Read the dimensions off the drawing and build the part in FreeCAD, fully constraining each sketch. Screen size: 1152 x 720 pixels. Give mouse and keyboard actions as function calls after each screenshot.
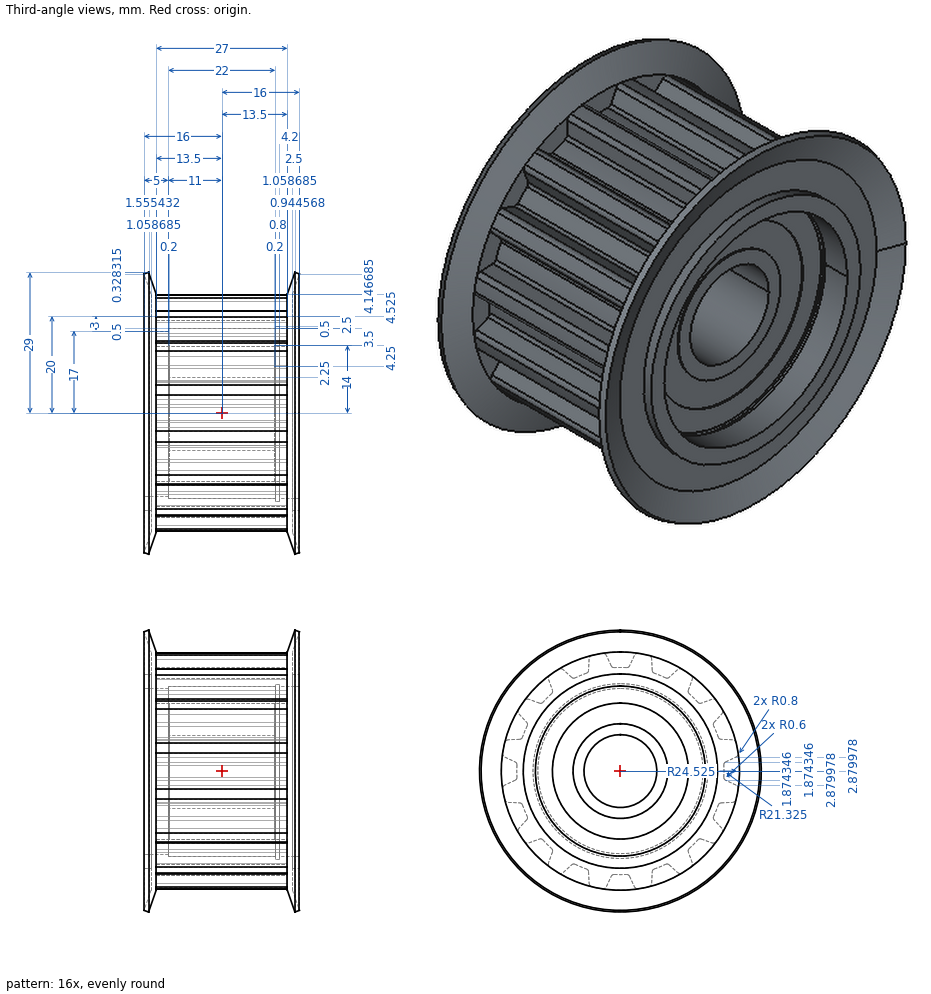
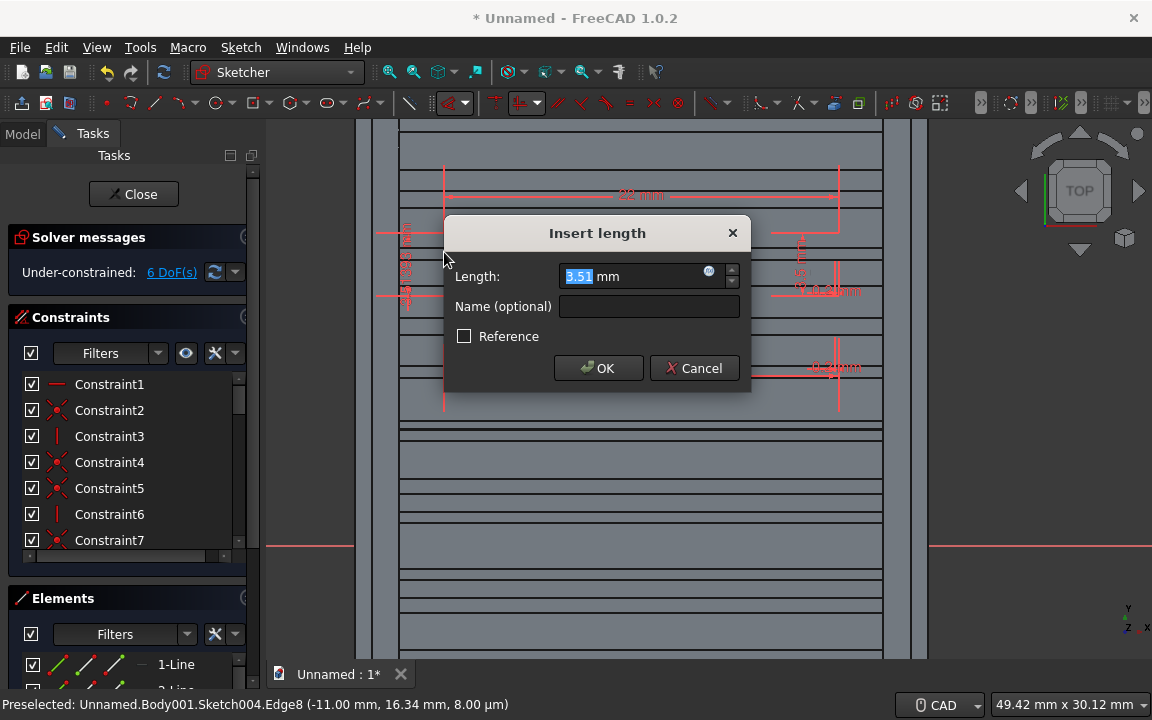
text(3.5)
key(Return)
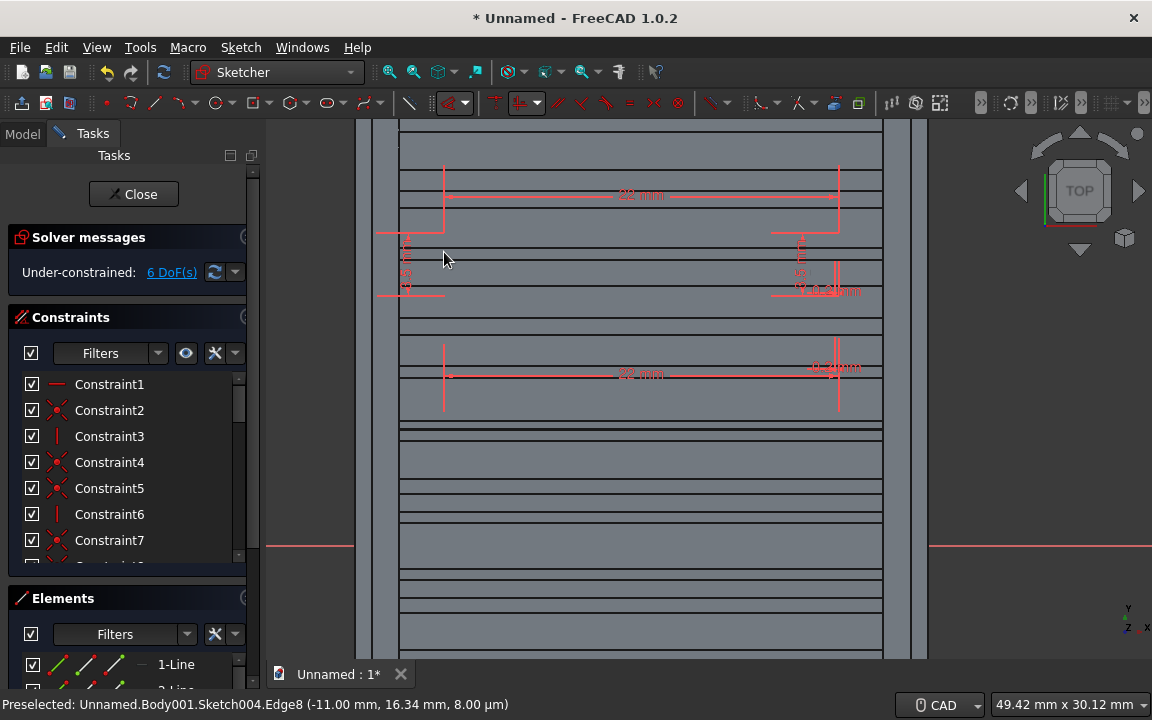
scroll(446, 296, up, 13)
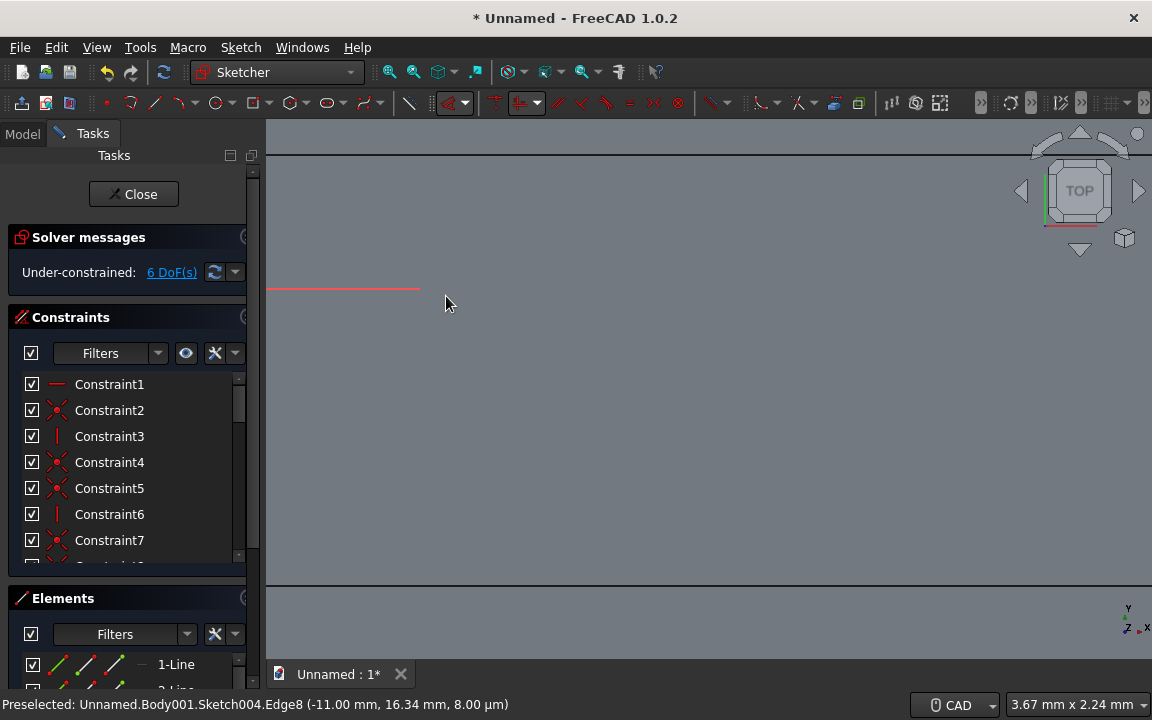
click(444, 289)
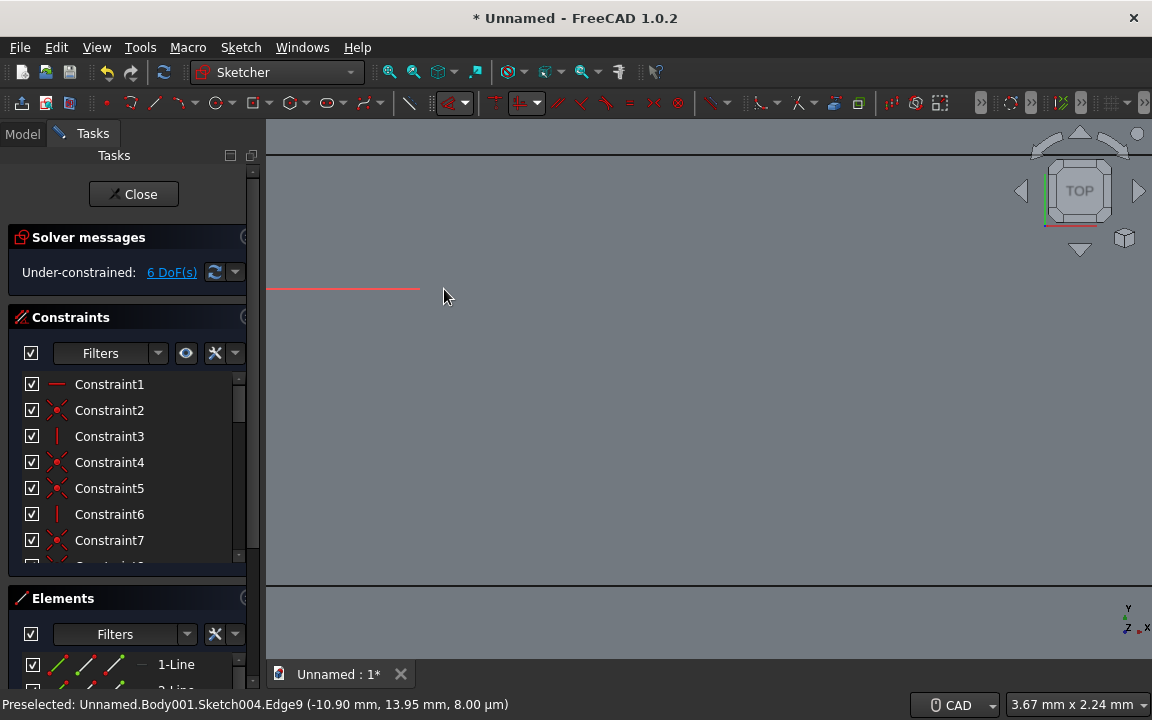
click(468, 104)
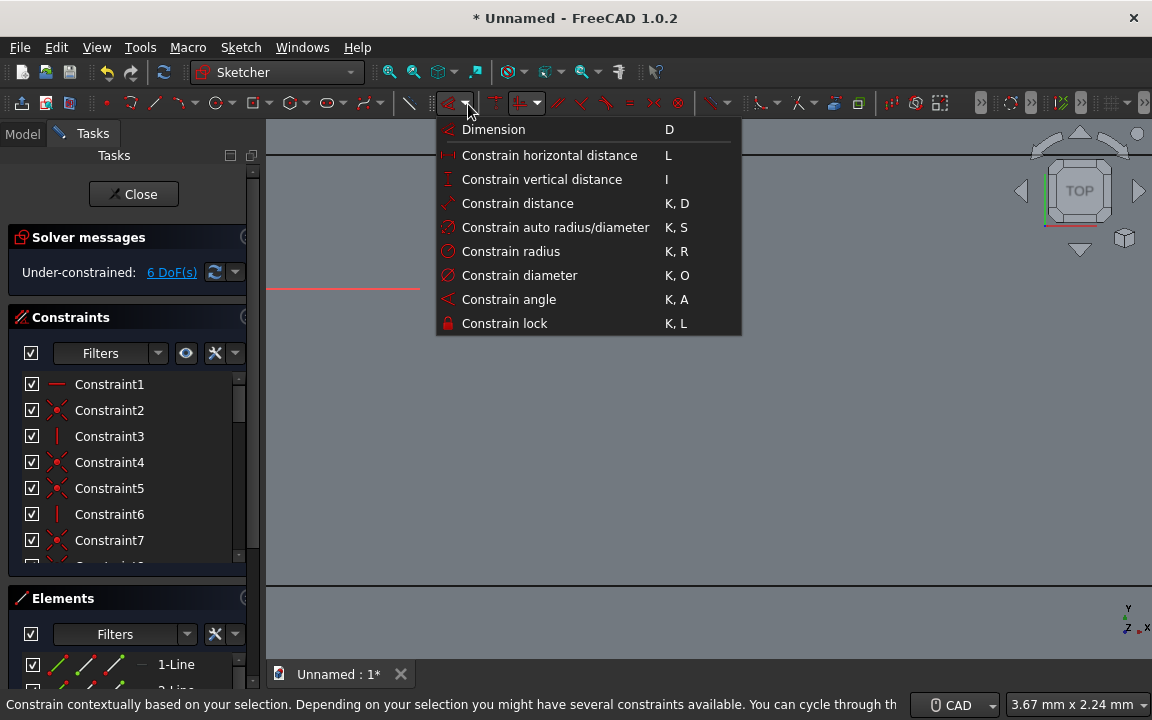
click(589, 155)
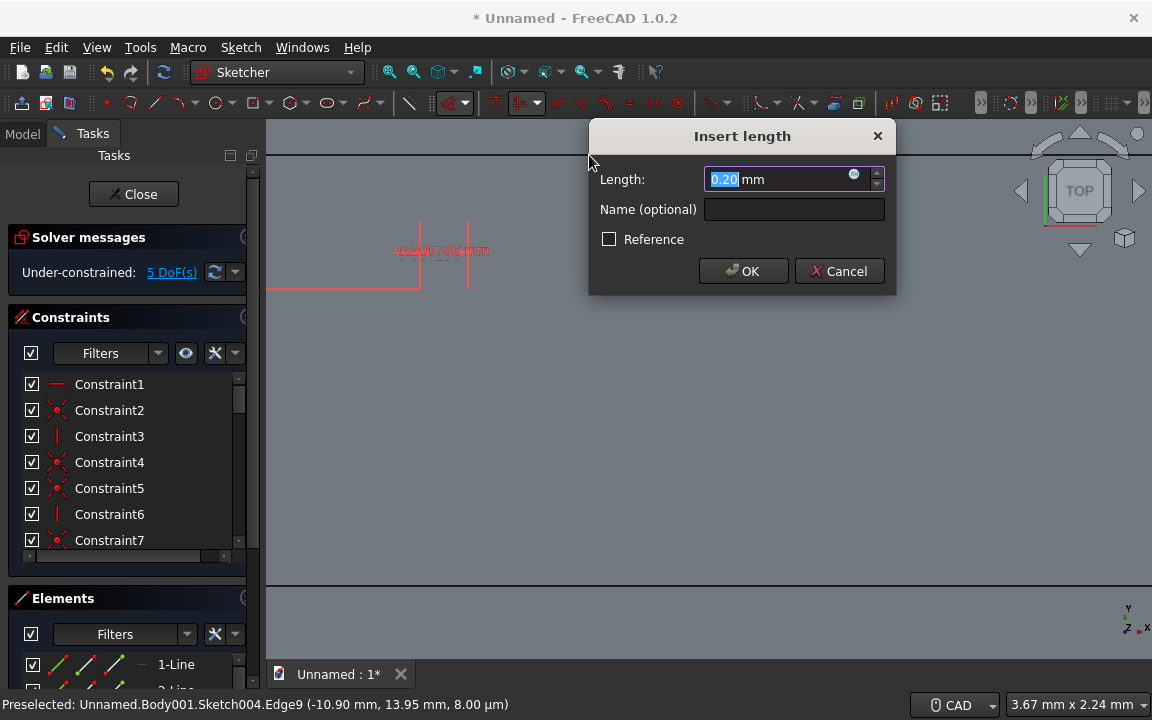
text(0.2)
key(Return)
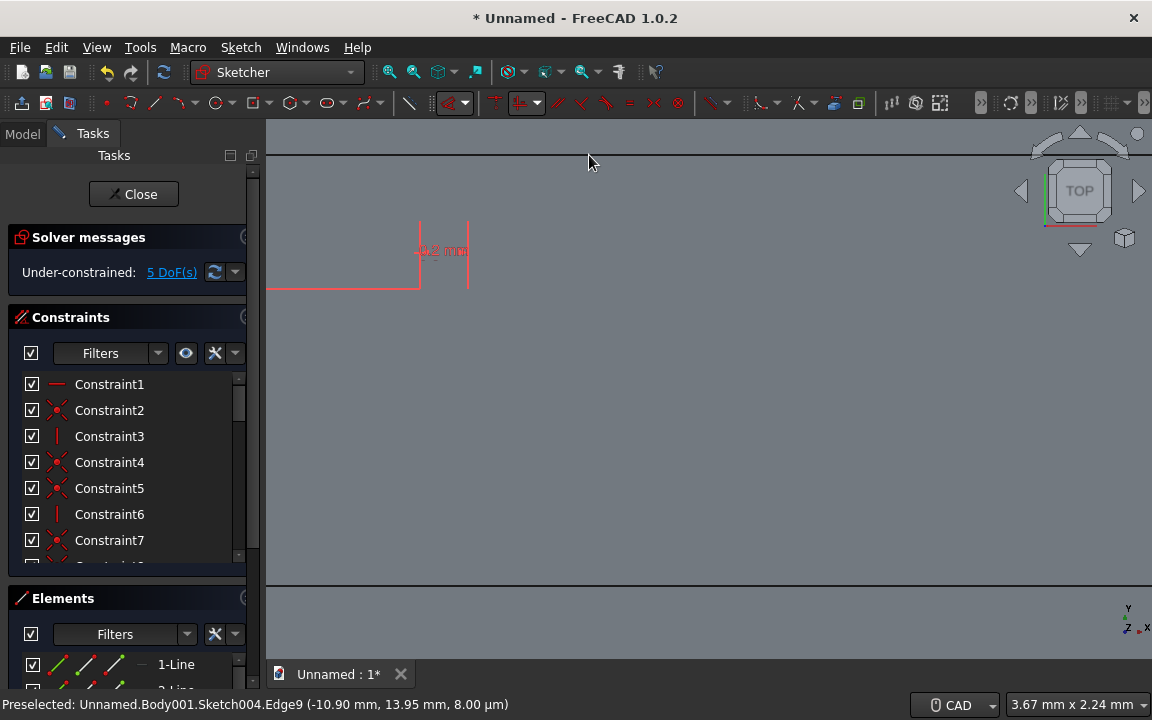
scroll(445, 296, down, 13)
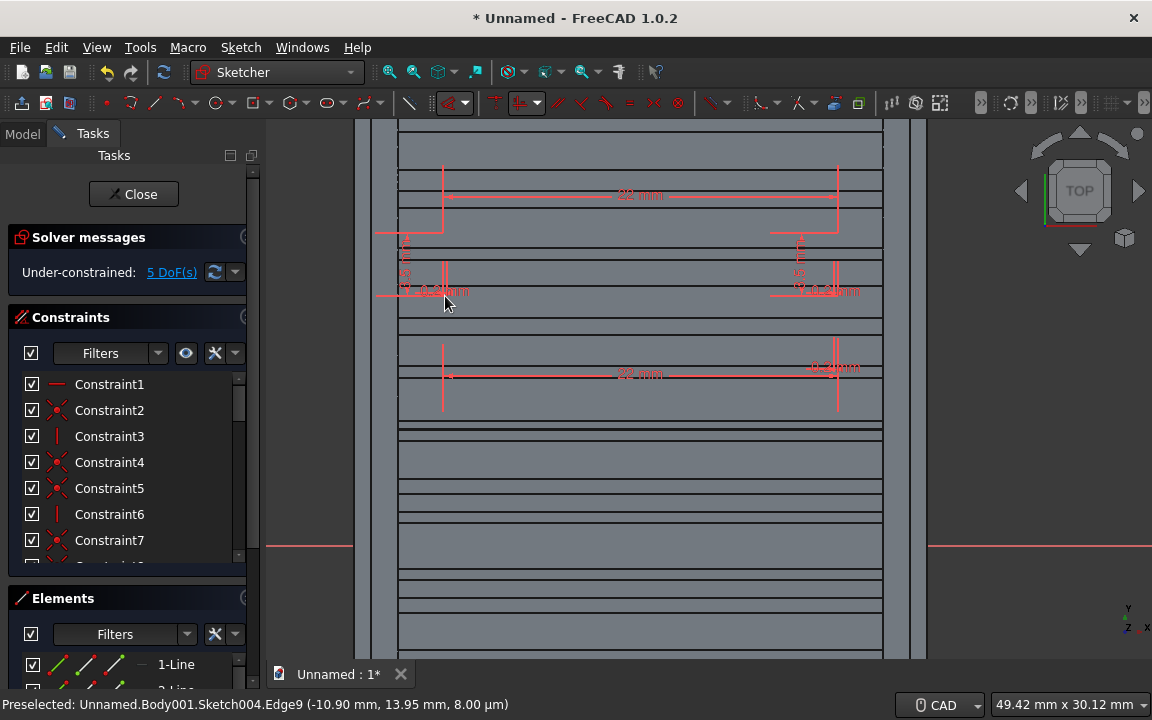
click(443, 412)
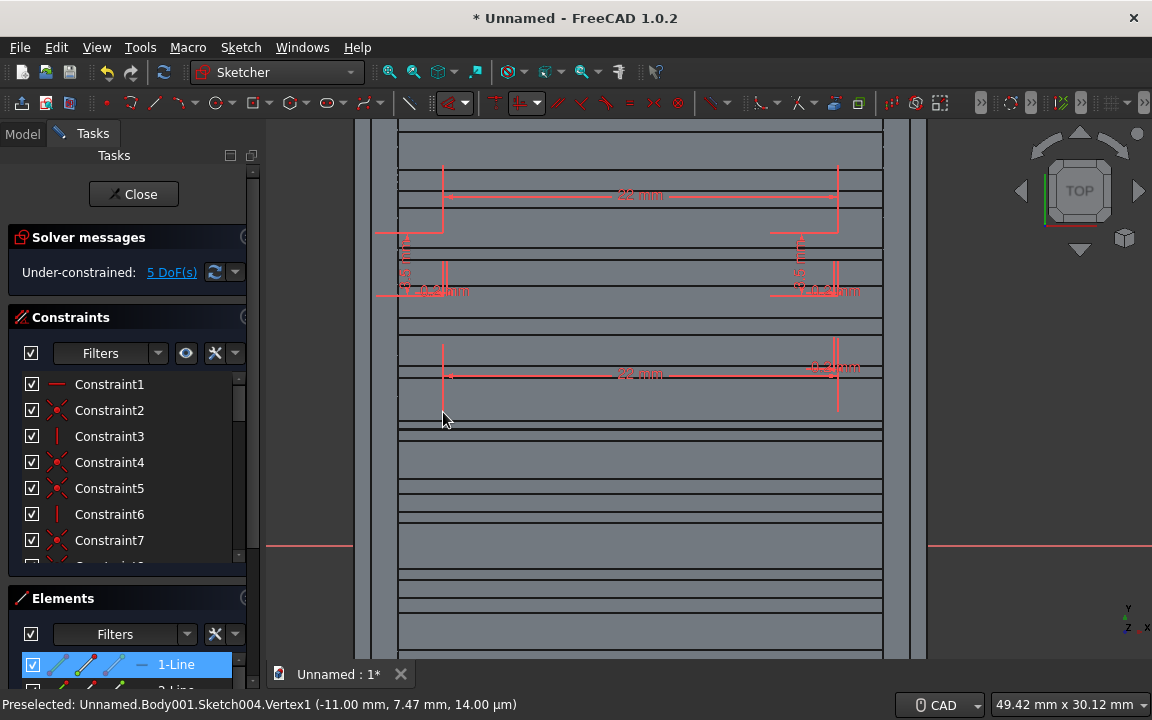
click(468, 104)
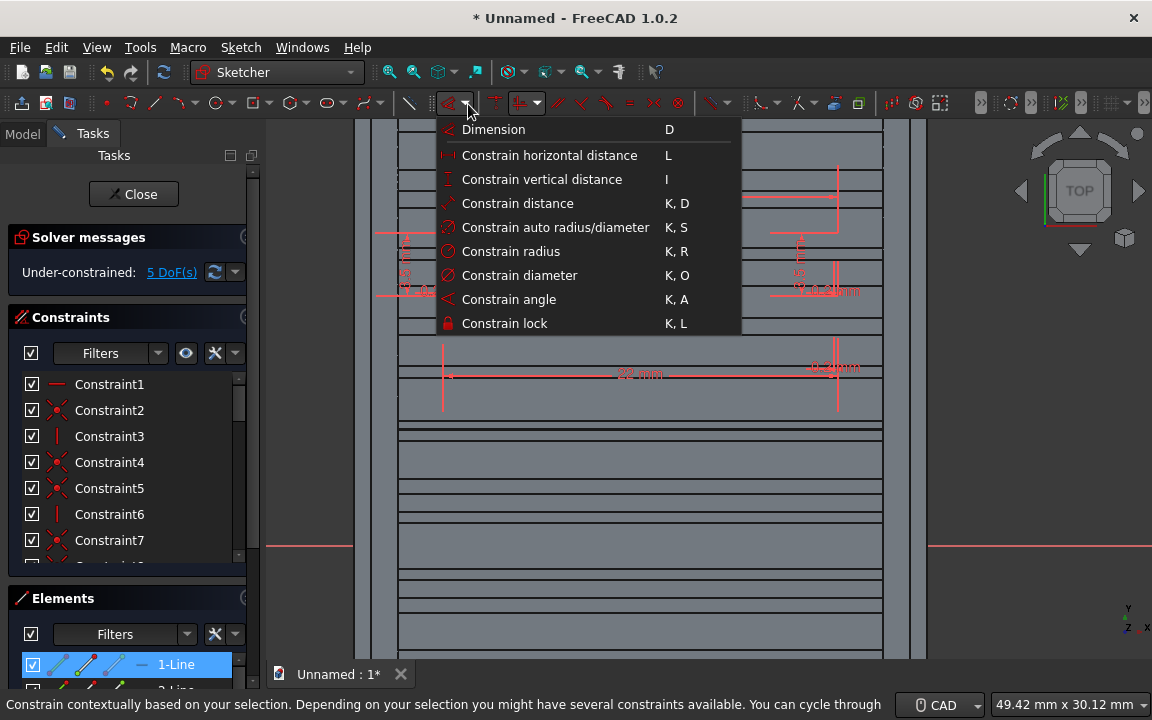
click(589, 155)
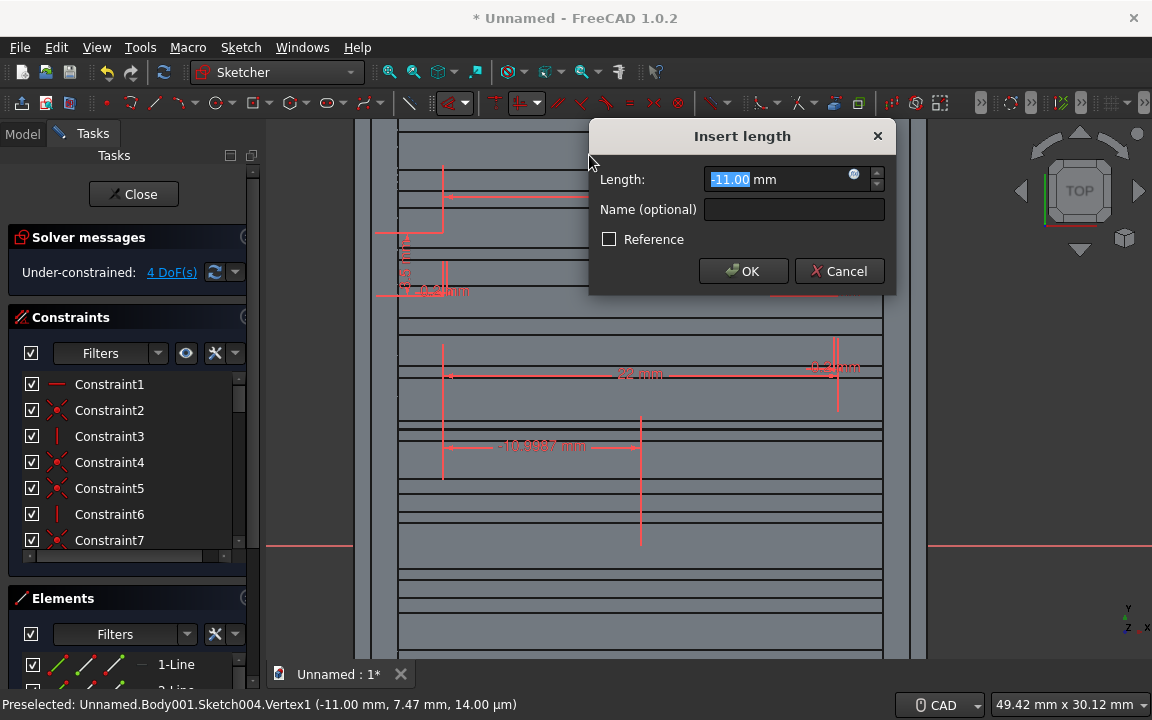
text(-11)
key(Return)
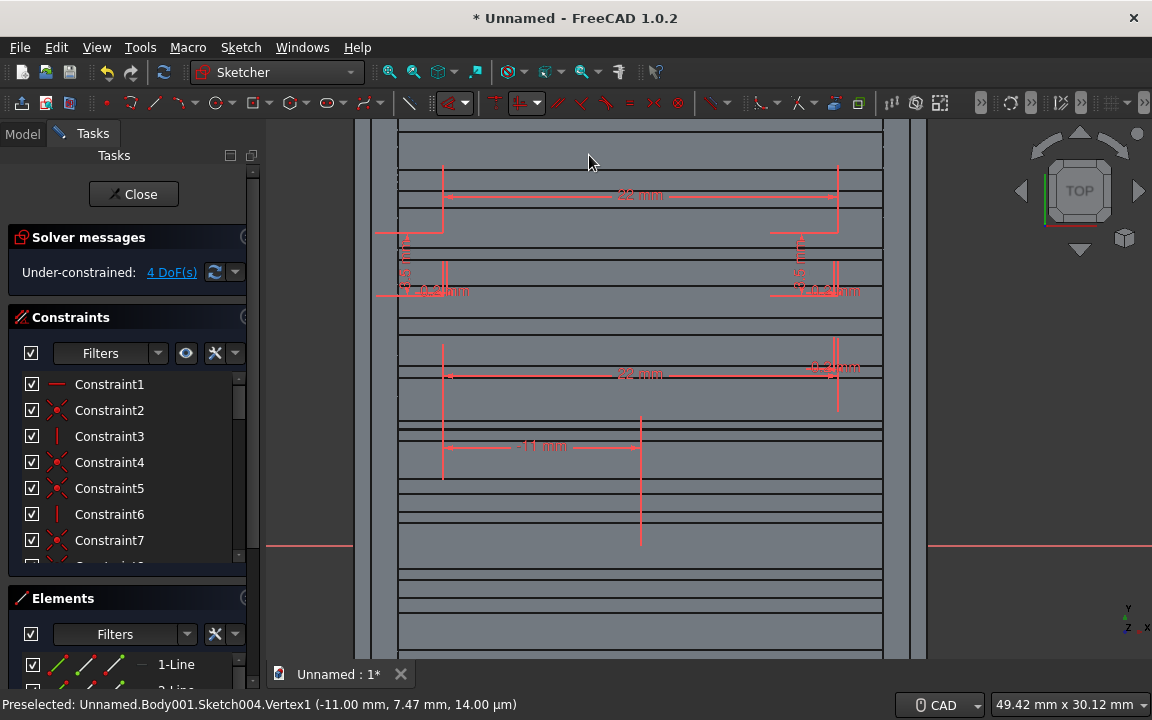
scroll(834, 296, up, 7)